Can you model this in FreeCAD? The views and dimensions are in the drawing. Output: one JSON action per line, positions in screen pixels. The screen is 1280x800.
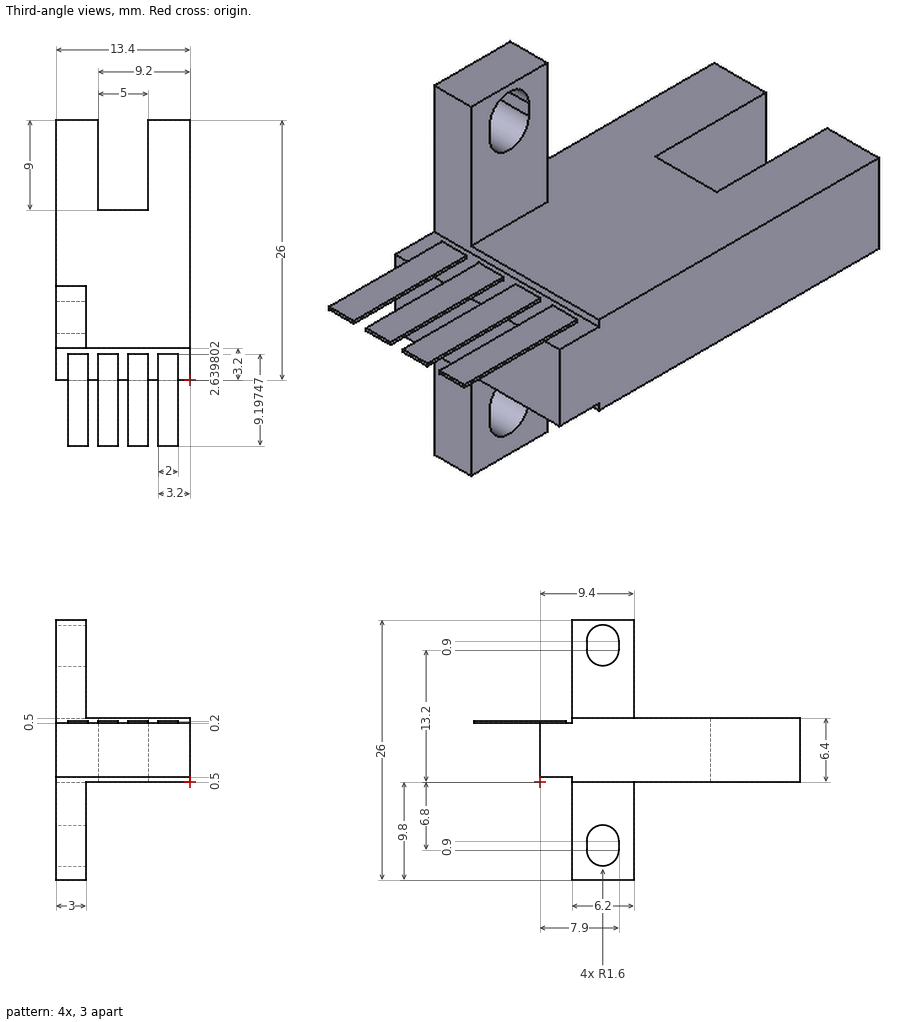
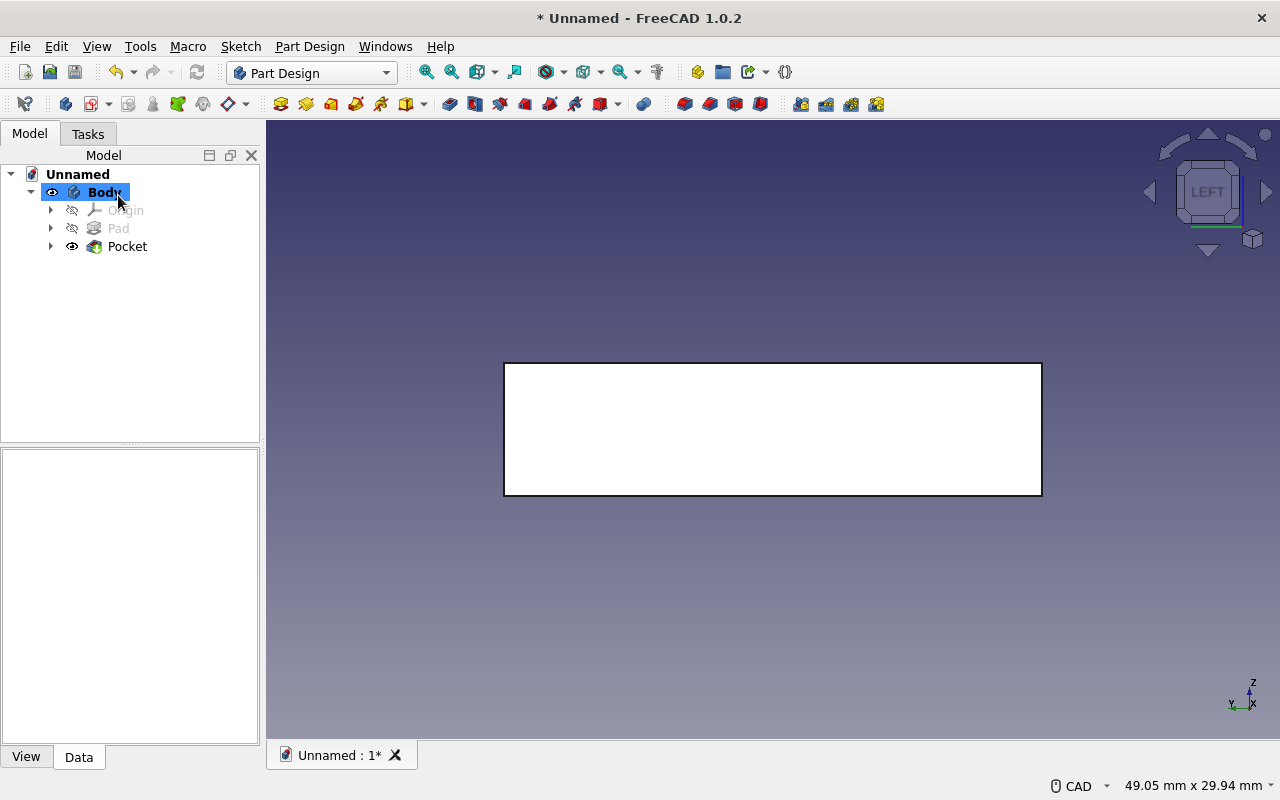
{"action": "left_click", "coordinate": [619, 428]}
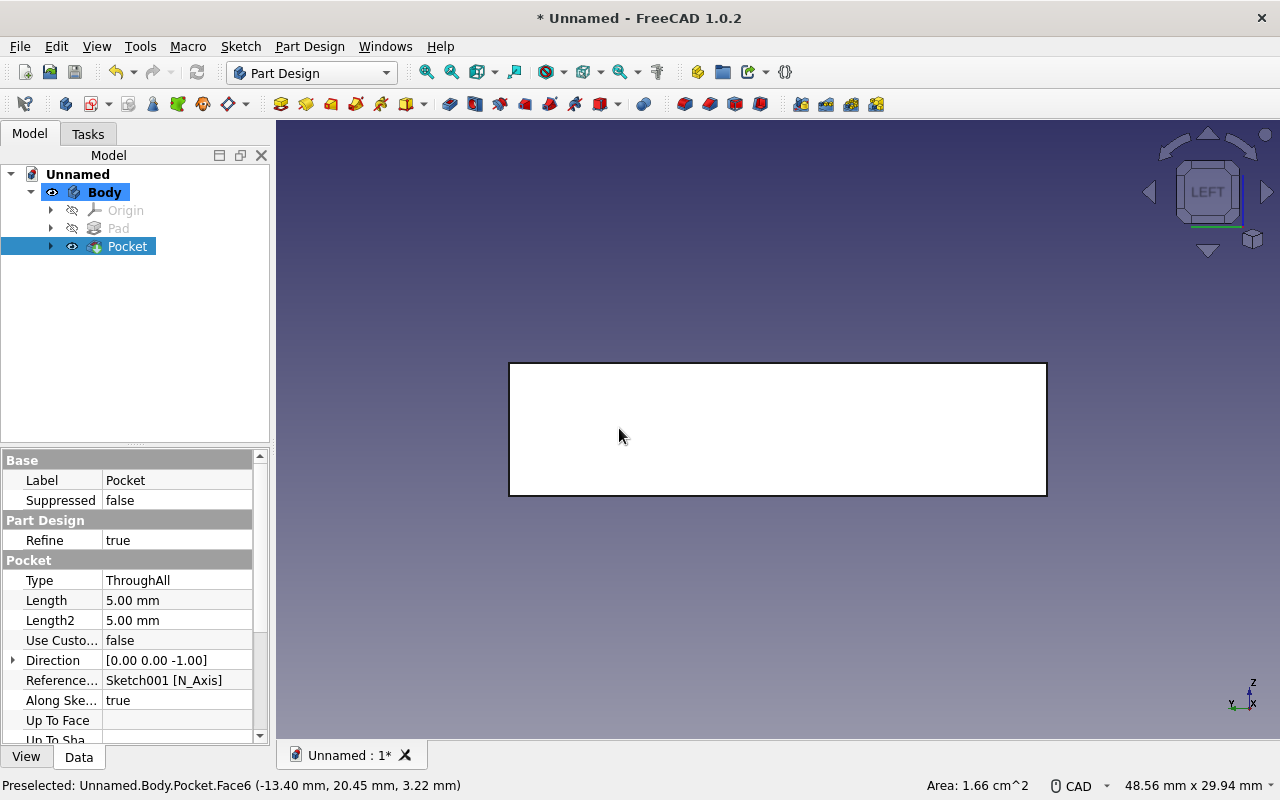
{"action": "left_click", "coordinate": [90, 104]}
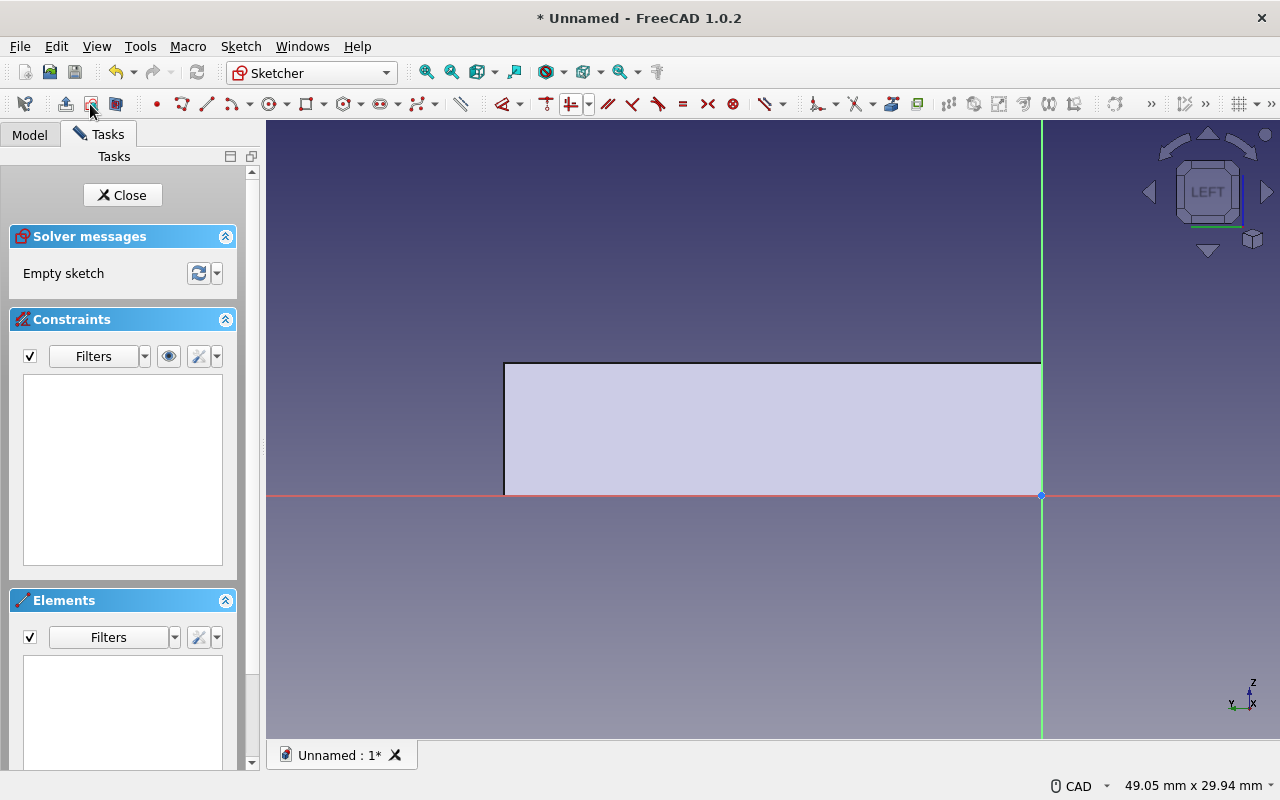
{"action": "scroll", "coordinate": [294, 430], "scroll_direction": "down", "scroll_amount": 2}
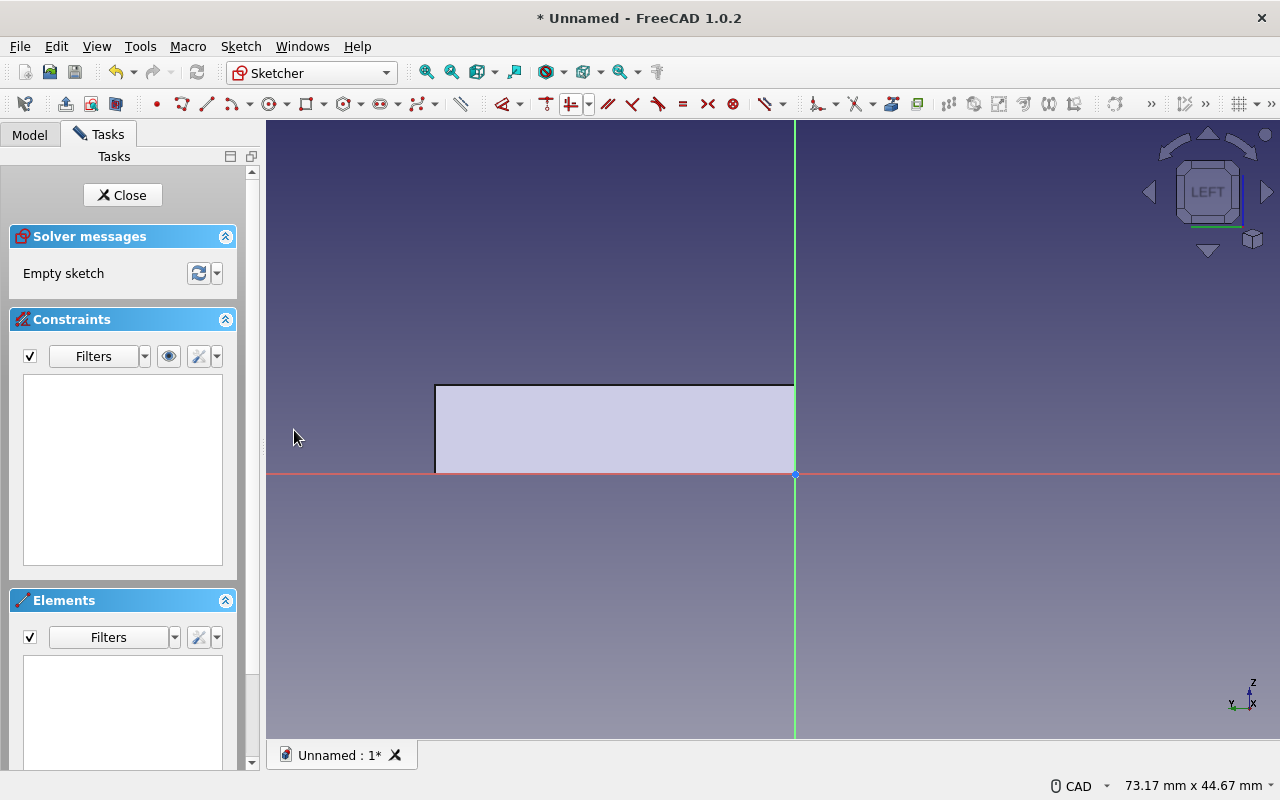
{"action": "left_click", "coordinate": [306, 104]}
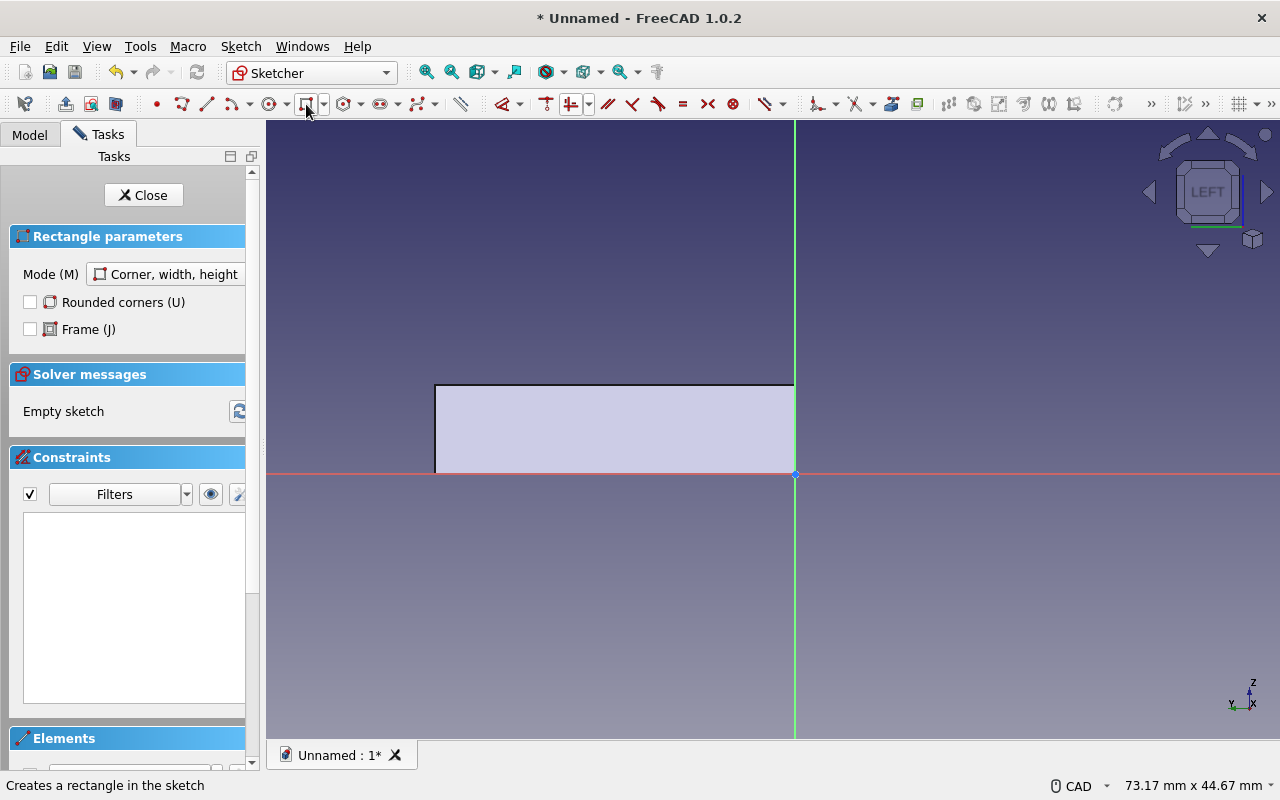
{"action": "left_click", "coordinate": [665, 250]}
{"action": "left_click", "coordinate": [751, 610]}
{"action": "key", "text": "Escape"}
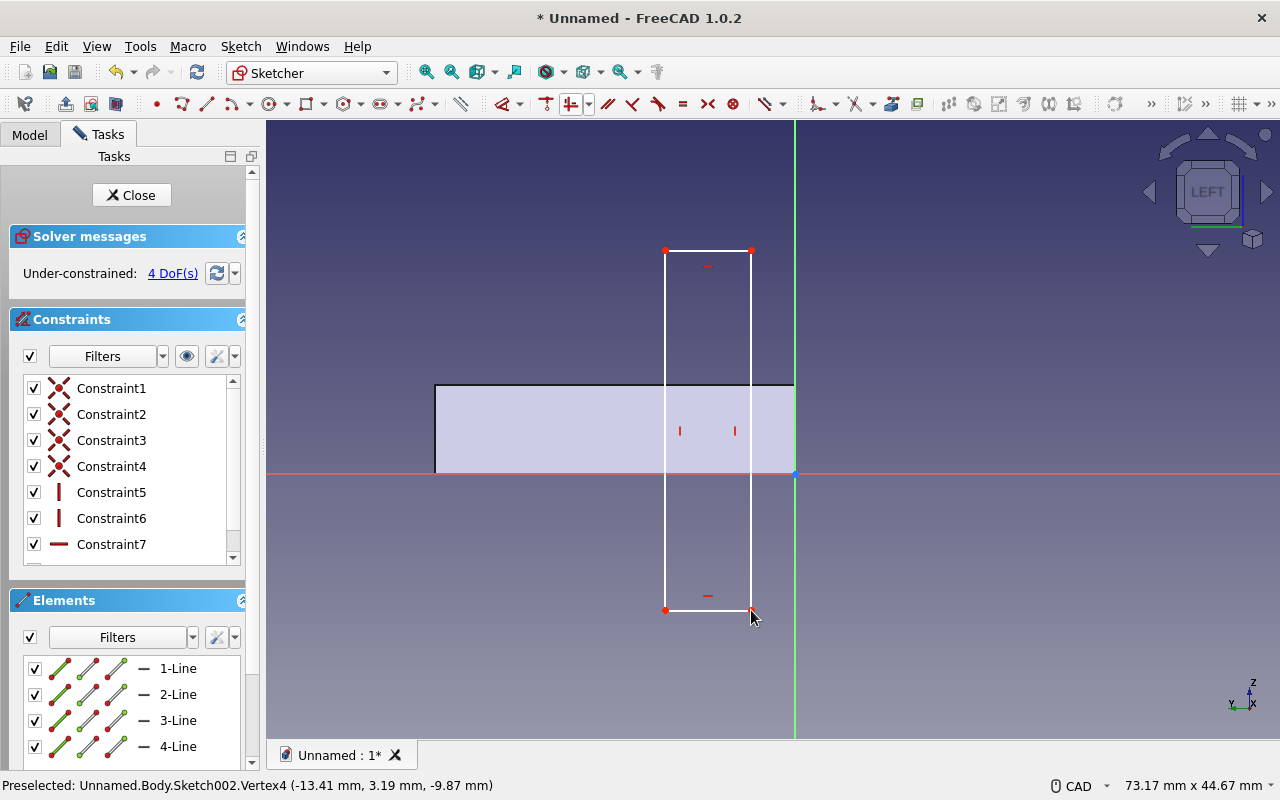
{"action": "left_click", "coordinate": [665, 359]}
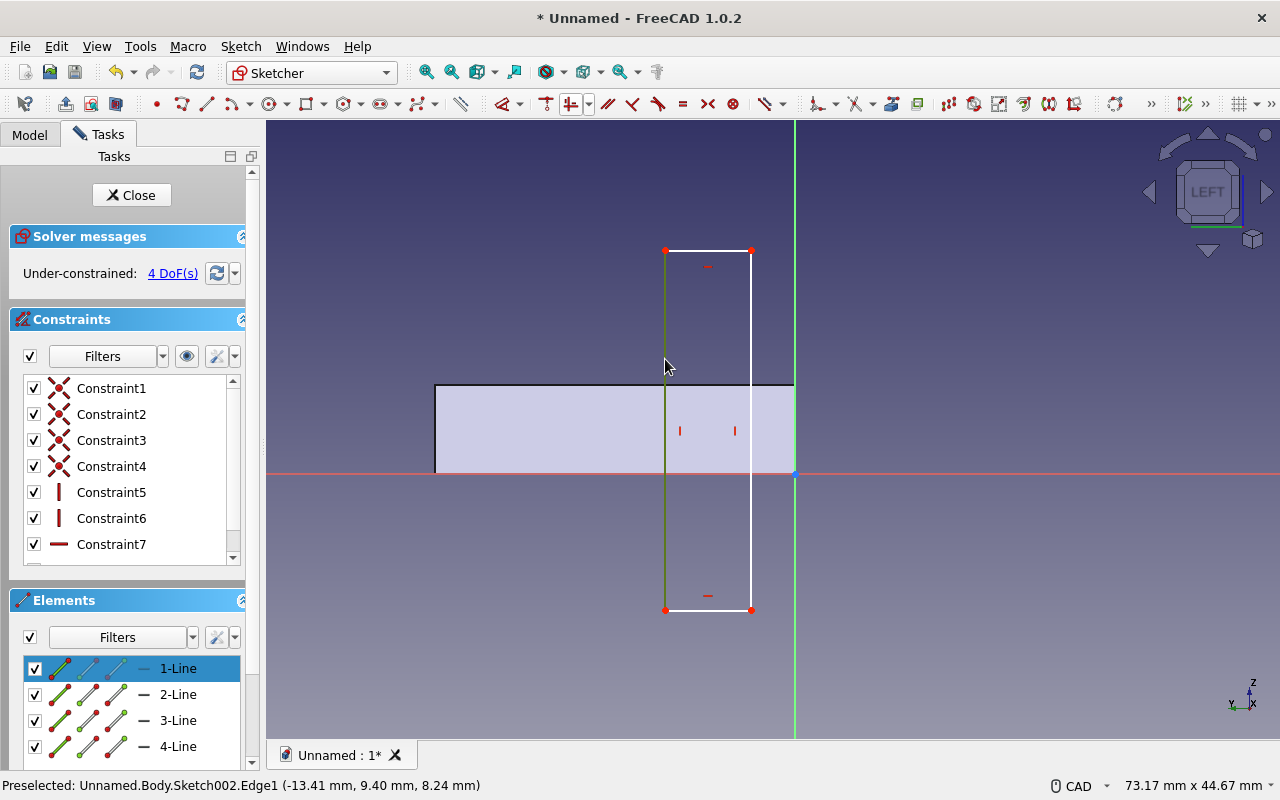
{"action": "key", "text": "i"}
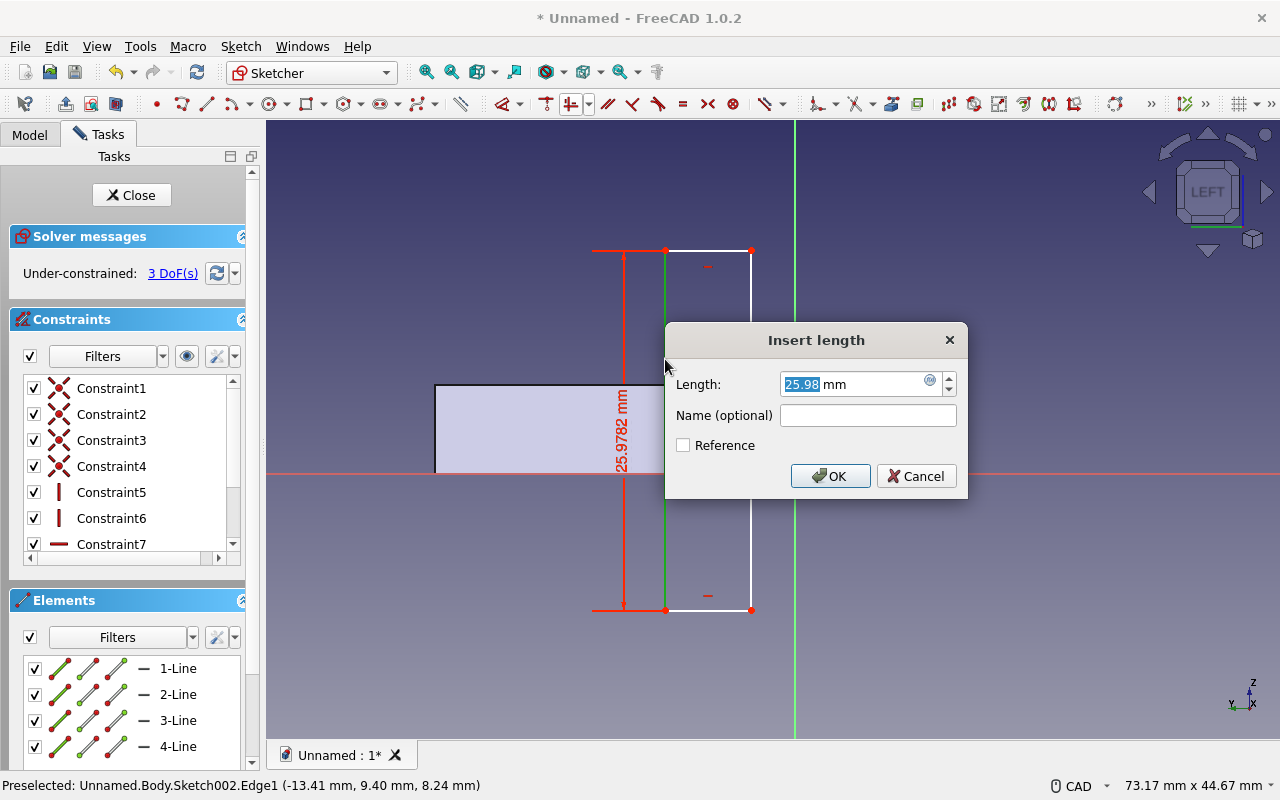
{"action": "type", "text": "26"}
{"action": "key", "text": "Return"}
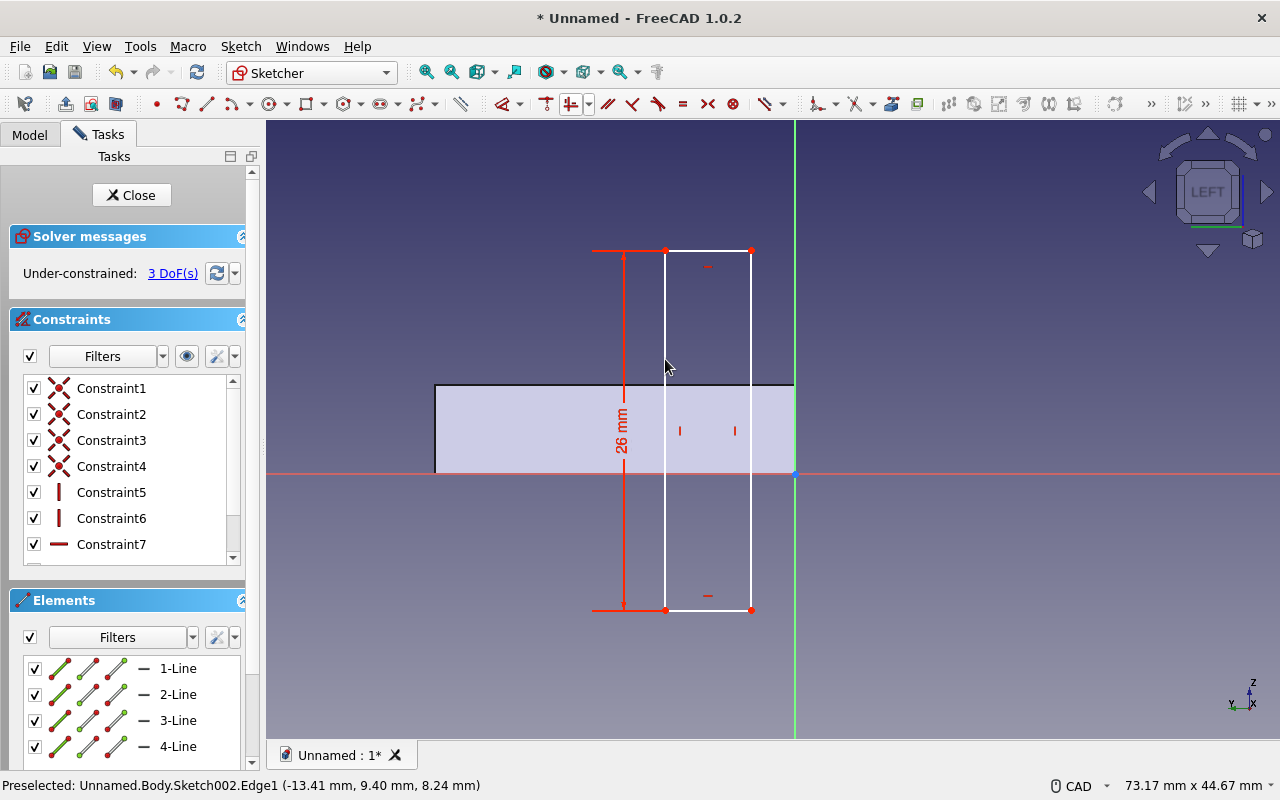
{"action": "left_click", "coordinate": [691, 611]}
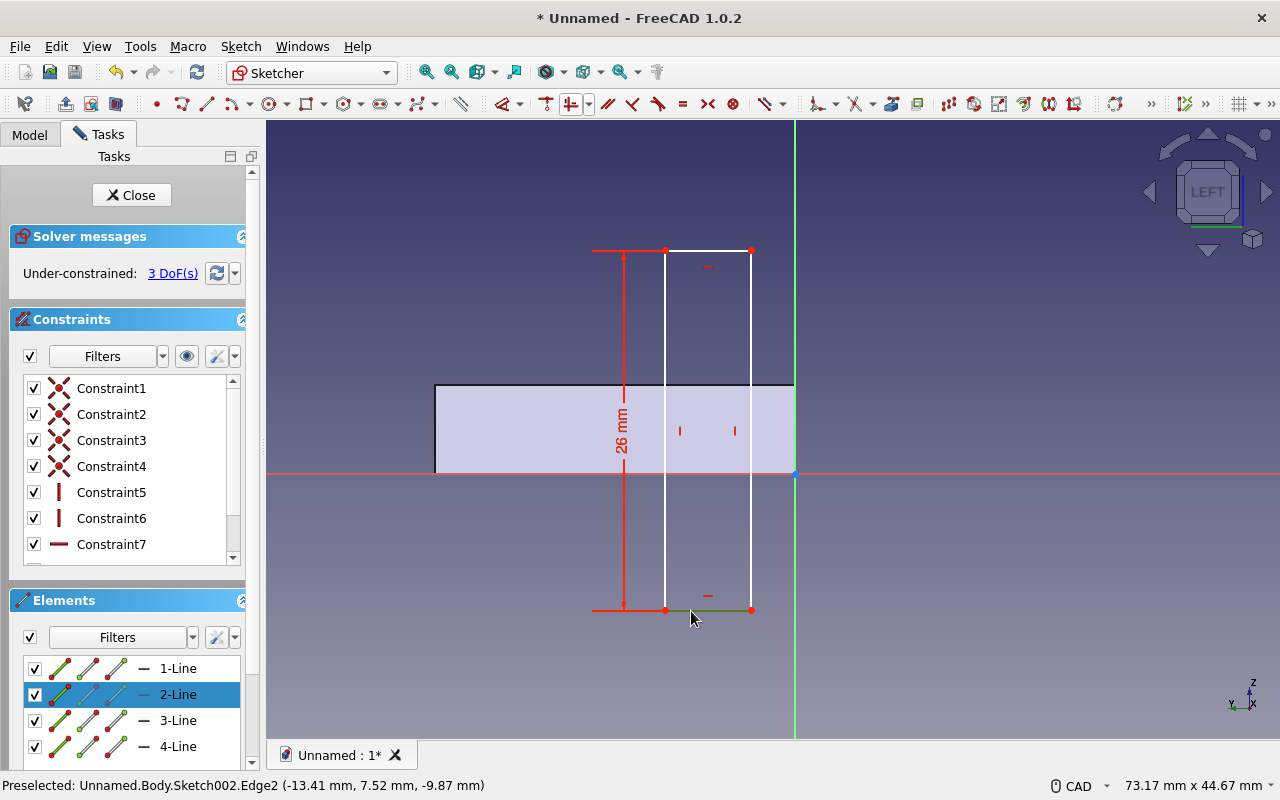
{"action": "key", "text": "l"}